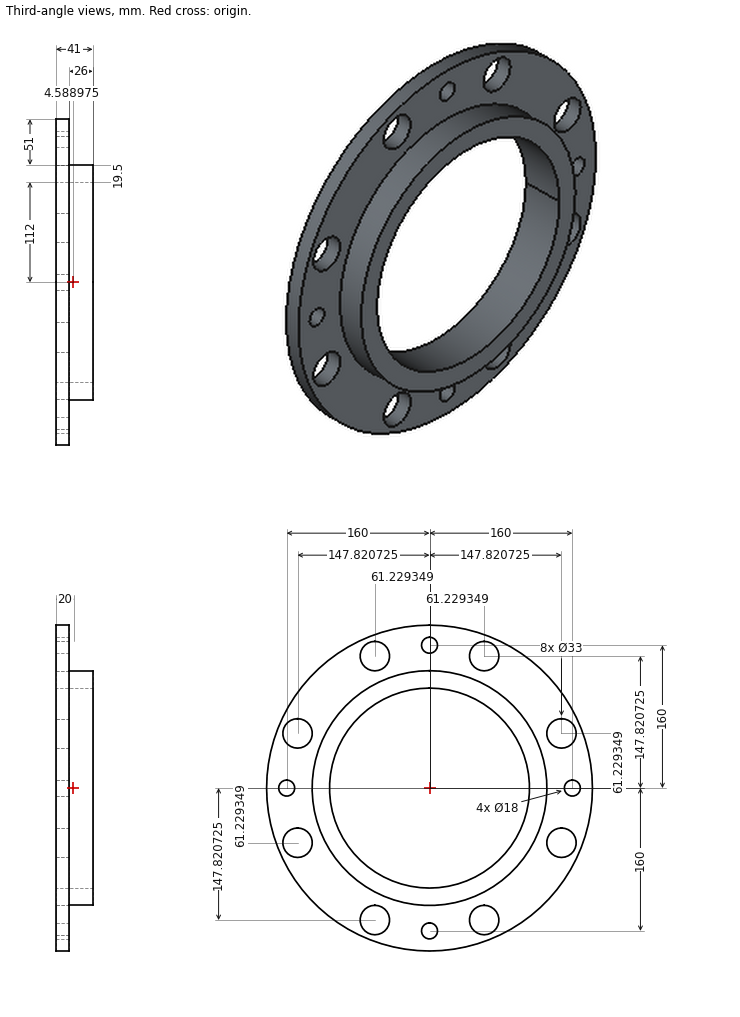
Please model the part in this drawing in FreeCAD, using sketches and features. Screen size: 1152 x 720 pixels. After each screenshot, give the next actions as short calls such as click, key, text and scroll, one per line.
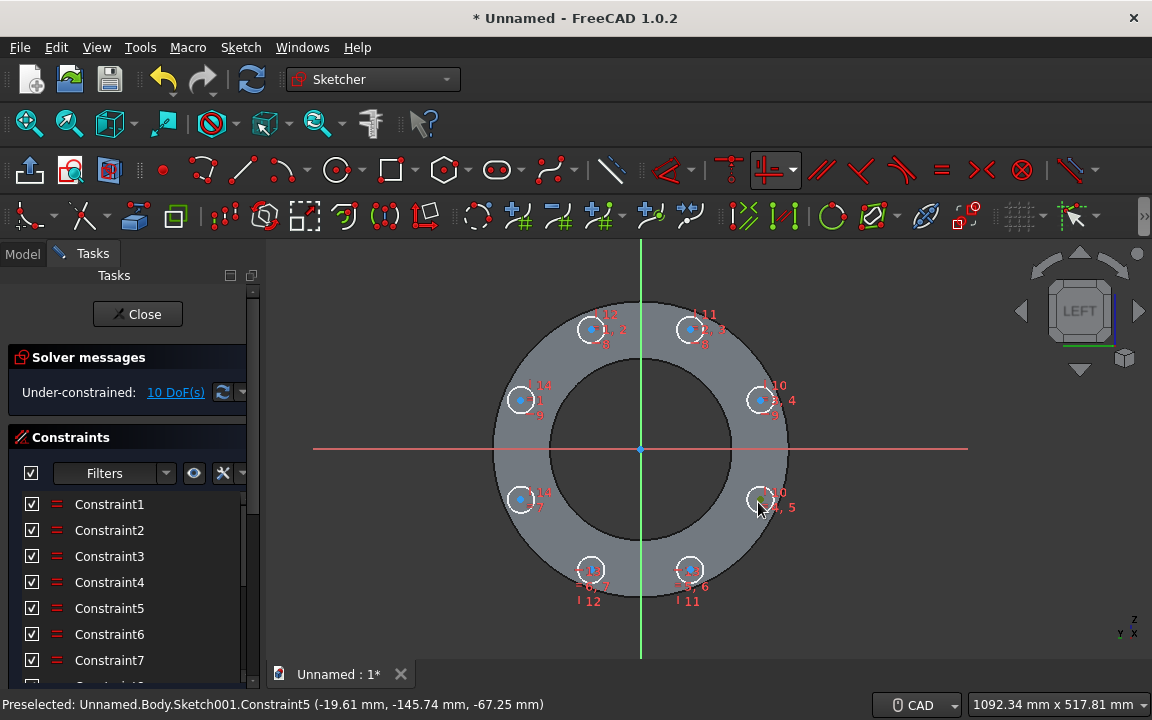
click(521, 500)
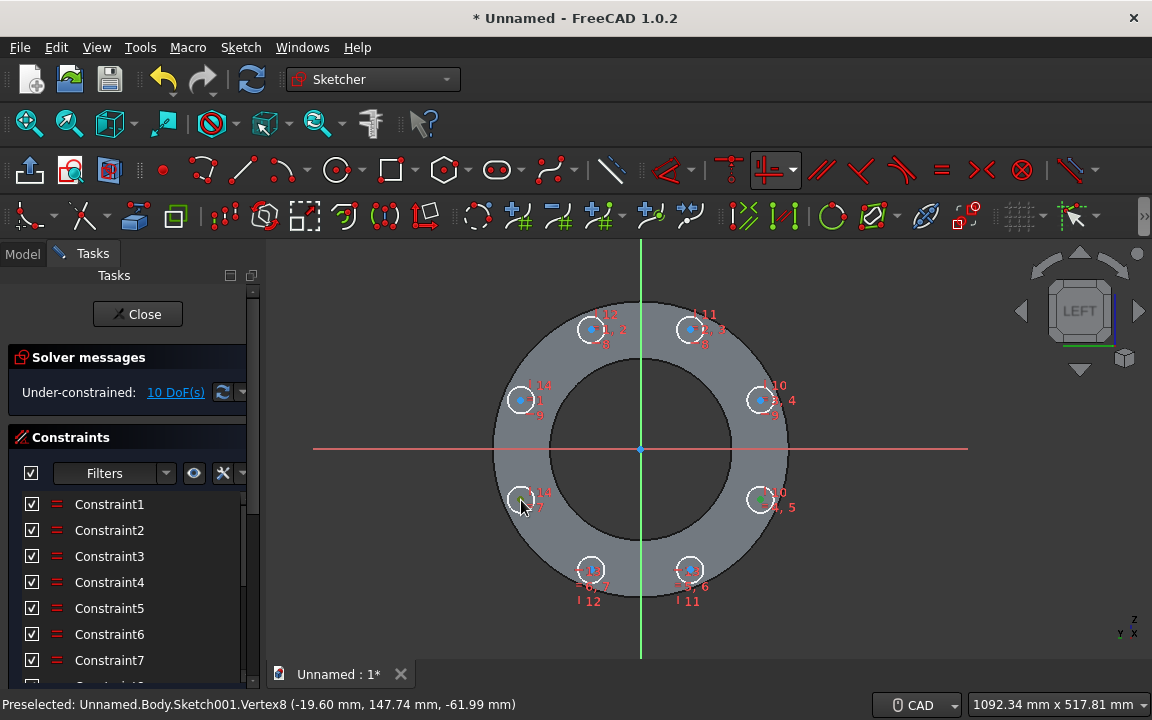
click(796, 170)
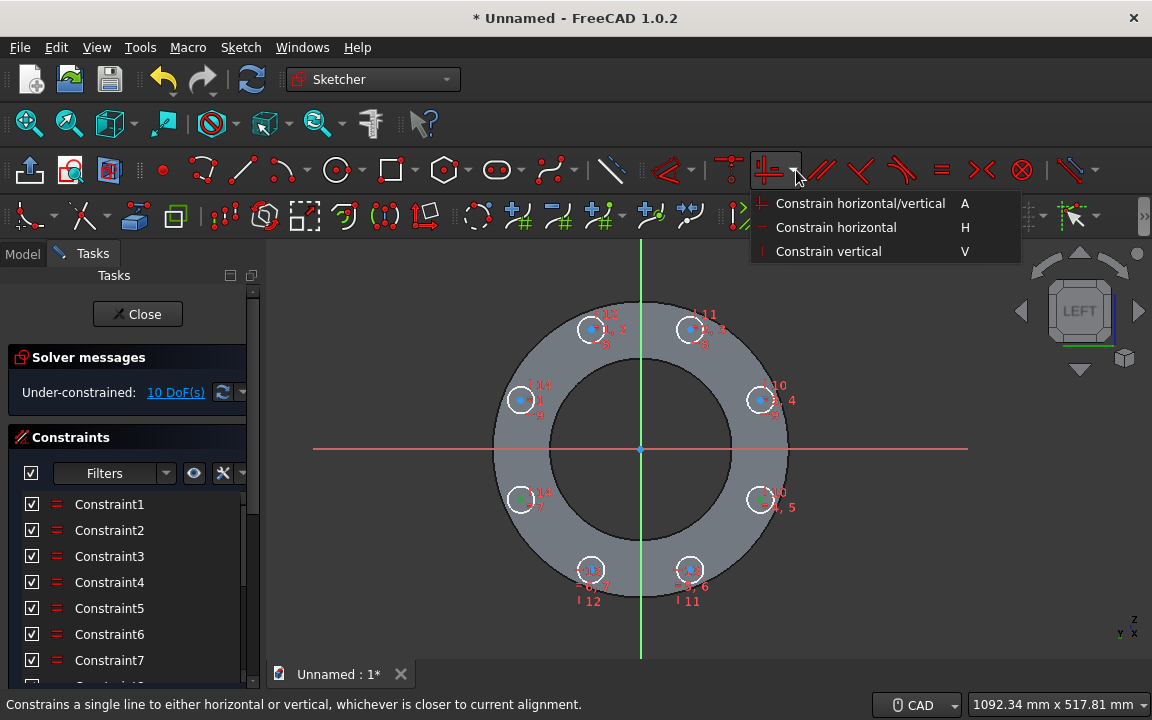
click(886, 227)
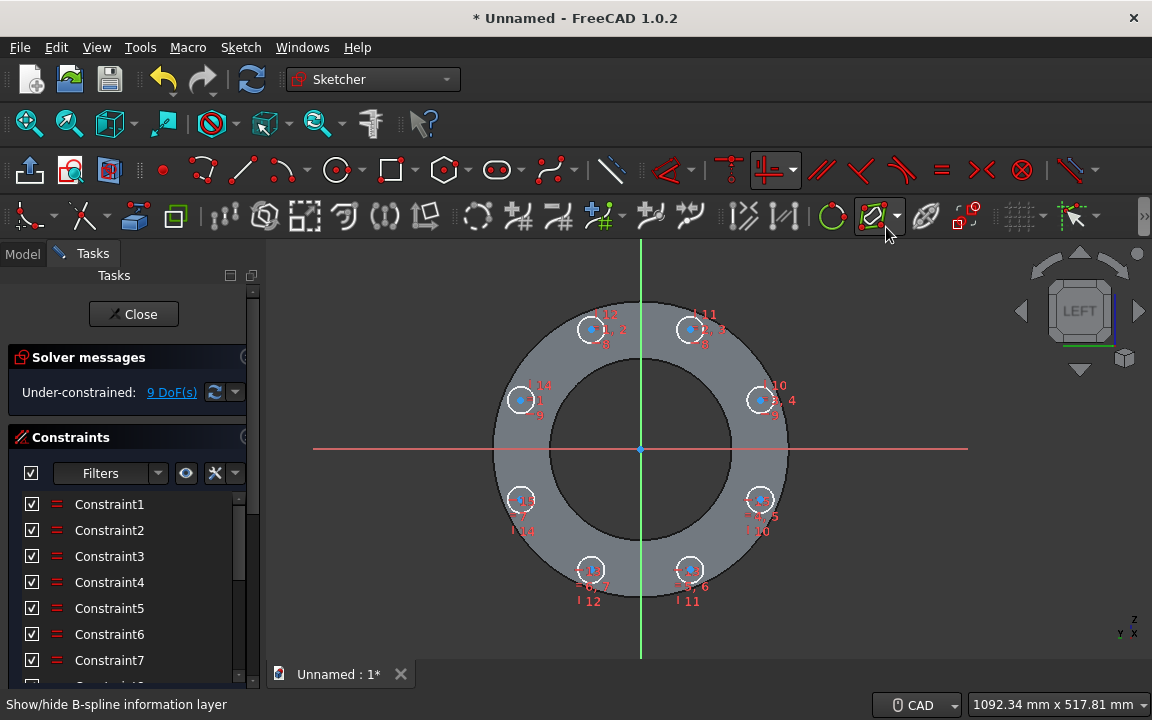
click(666, 170)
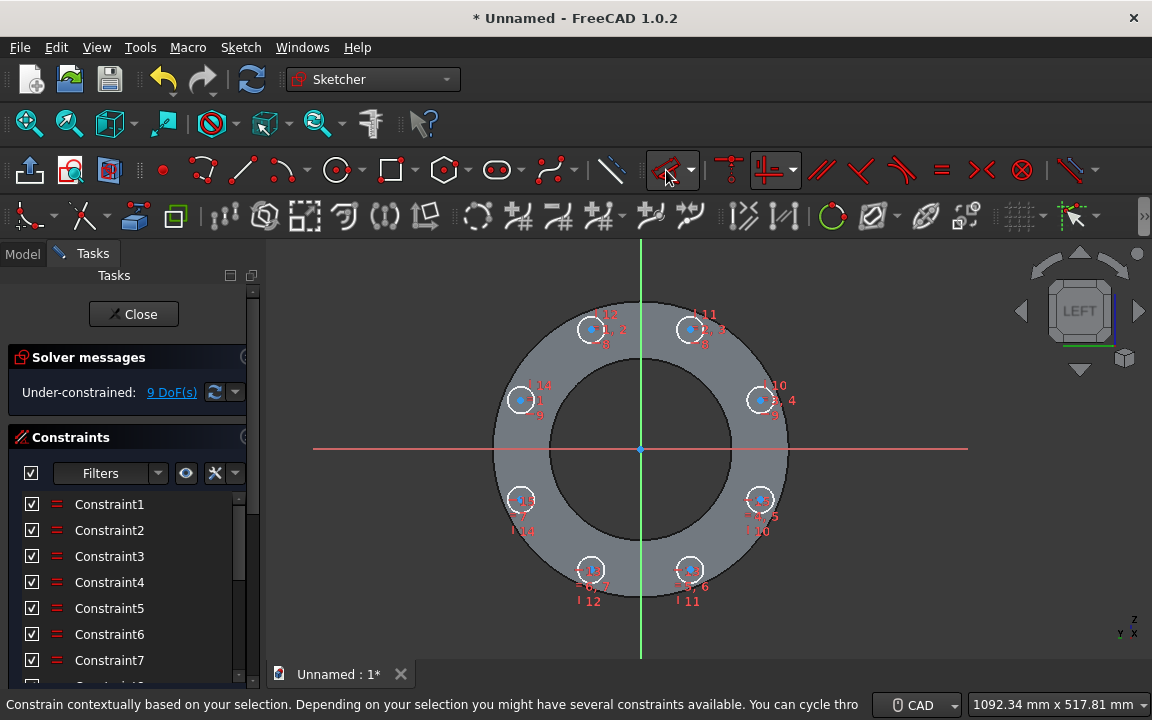
scroll(530, 391, up, 2)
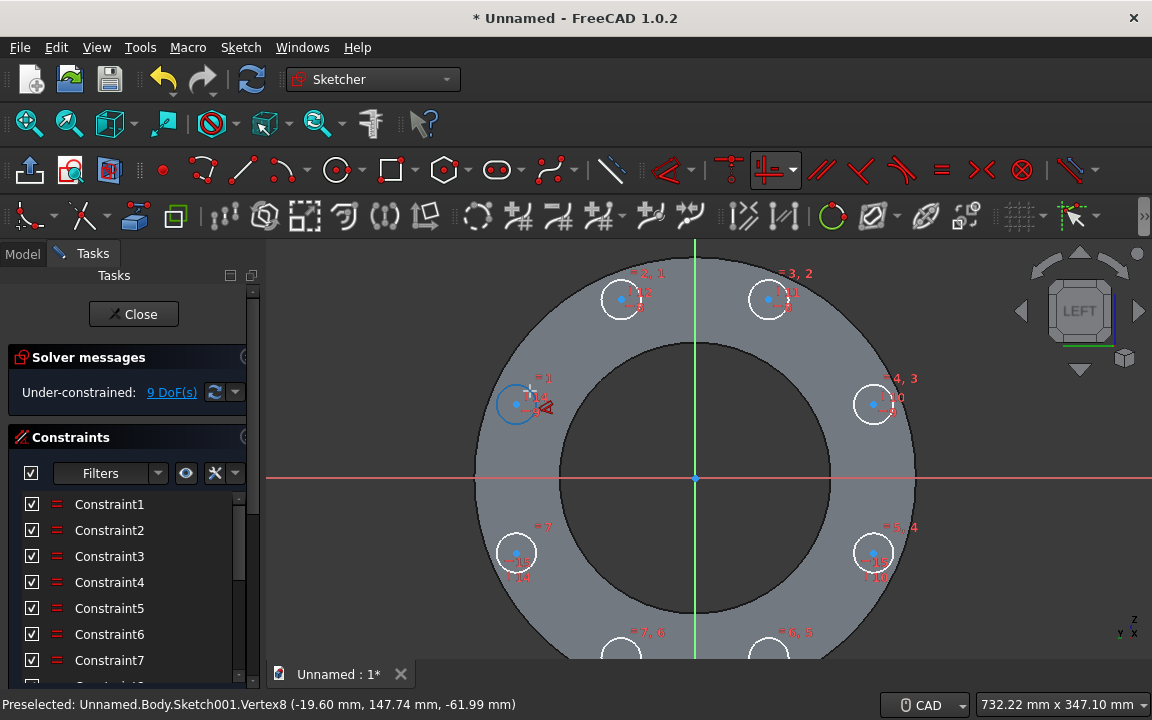
click(530, 391)
click(553, 368)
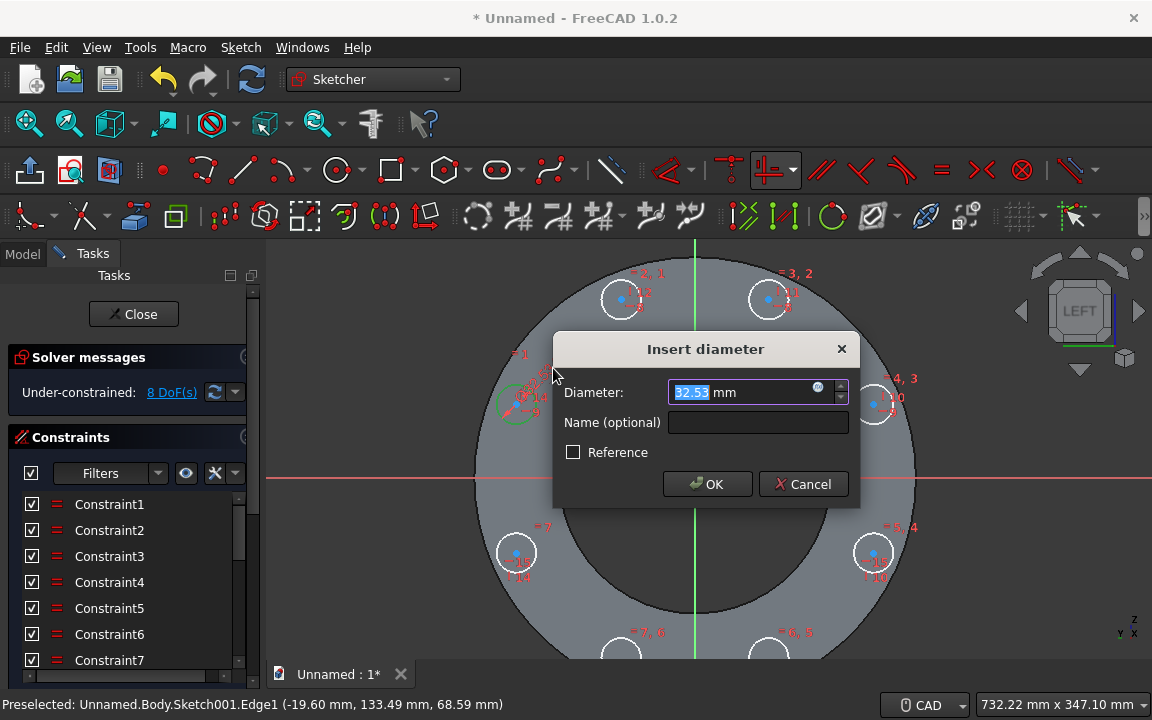
text(33)
key(Return)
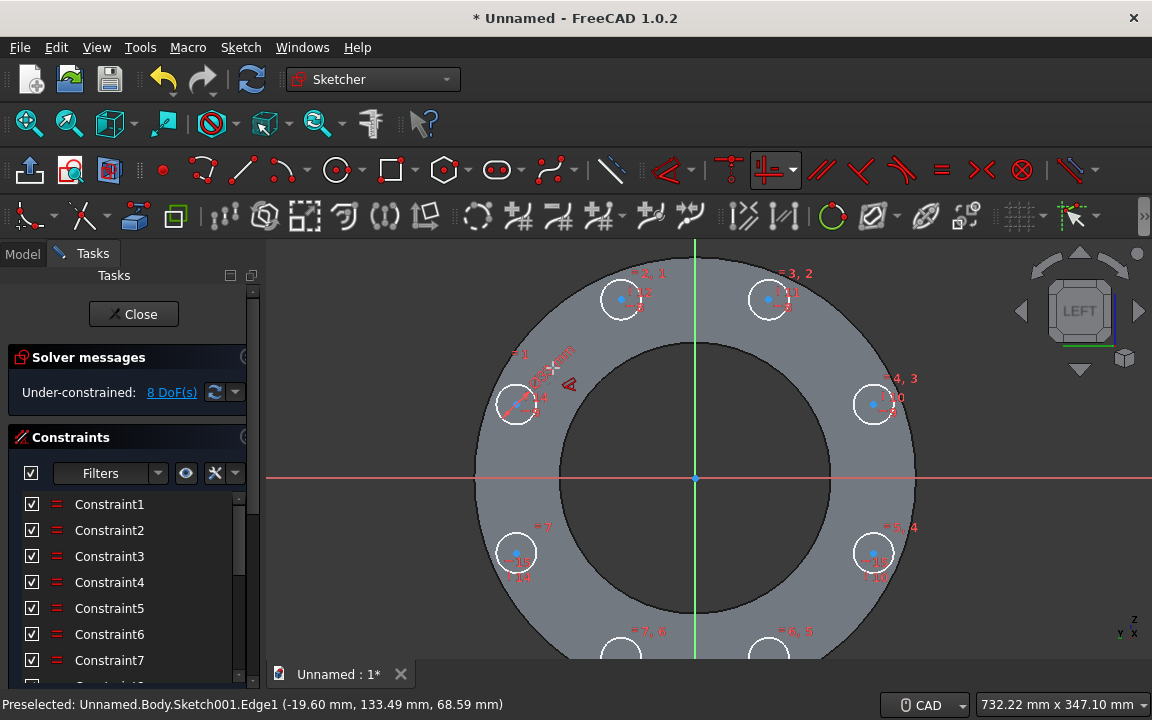
click(516, 405)
click(482, 441)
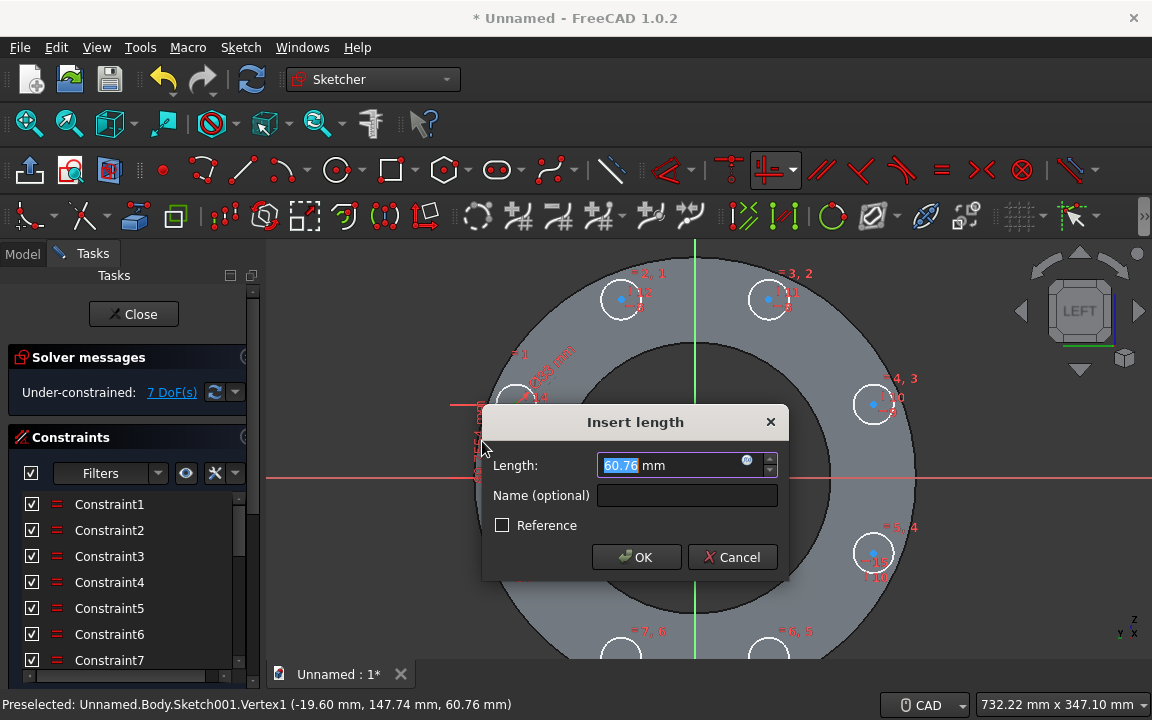
text(61.229349)
key(Return)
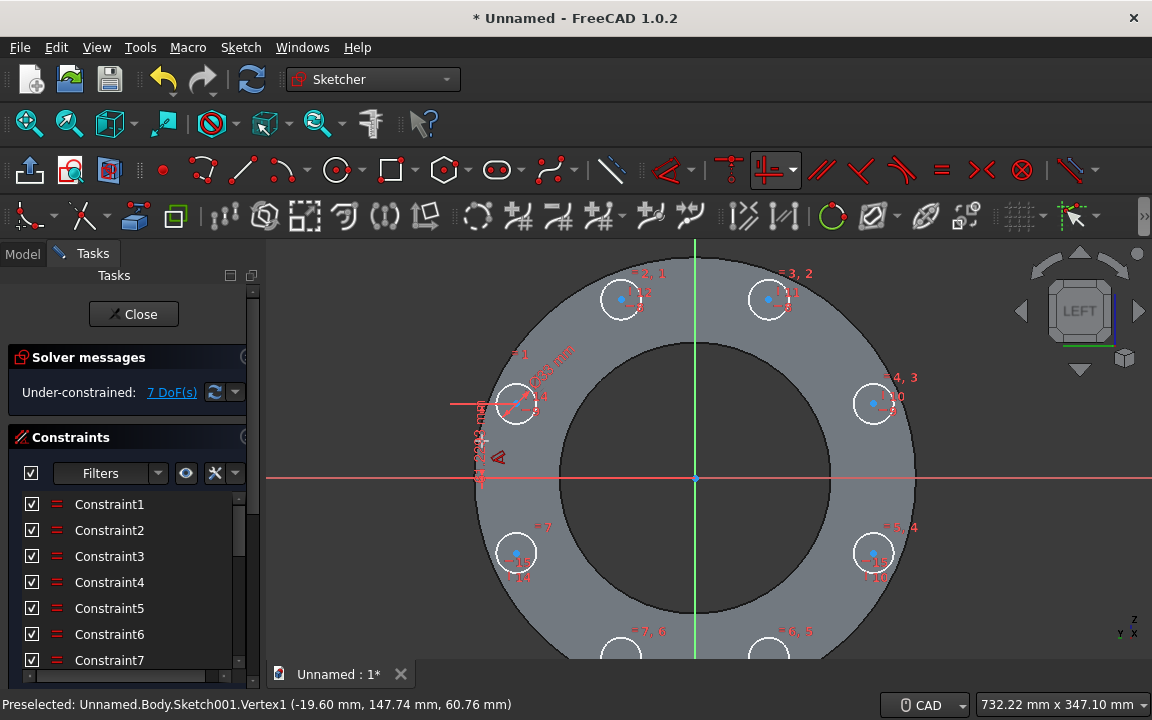
click(621, 300)
click(658, 512)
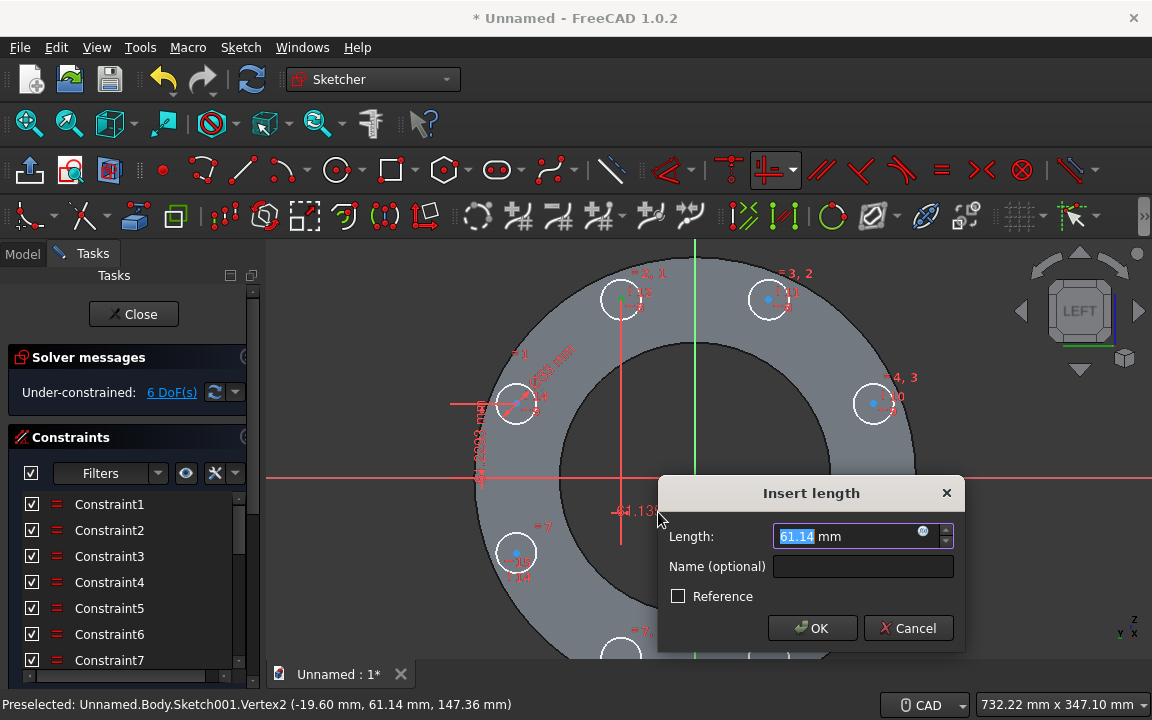
text(61.229349)
key(Return)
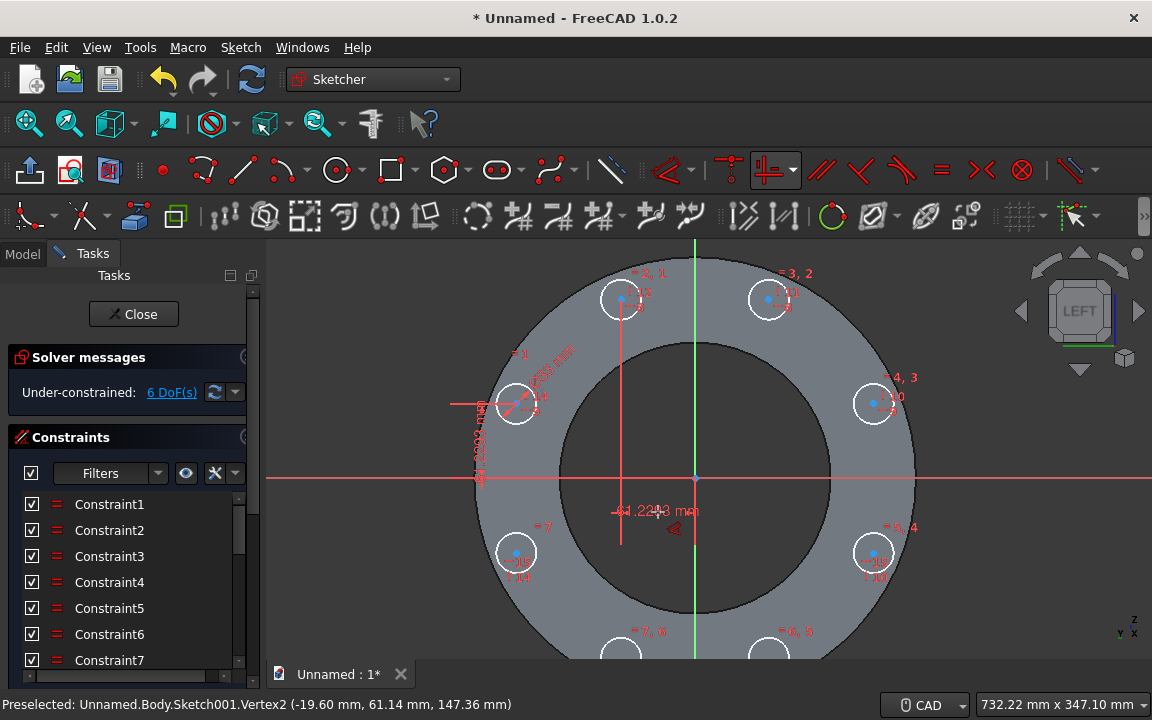
click(769, 300)
click(732, 512)